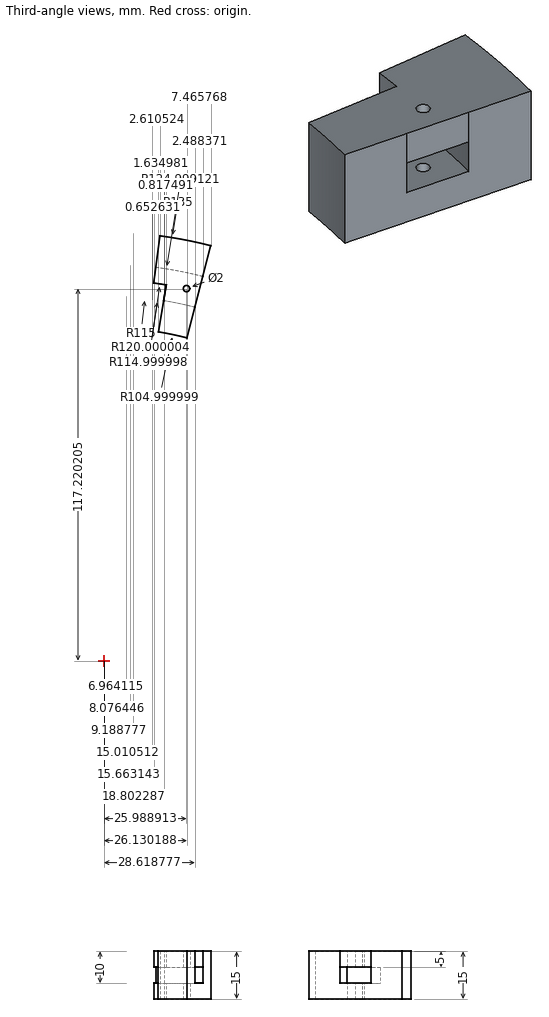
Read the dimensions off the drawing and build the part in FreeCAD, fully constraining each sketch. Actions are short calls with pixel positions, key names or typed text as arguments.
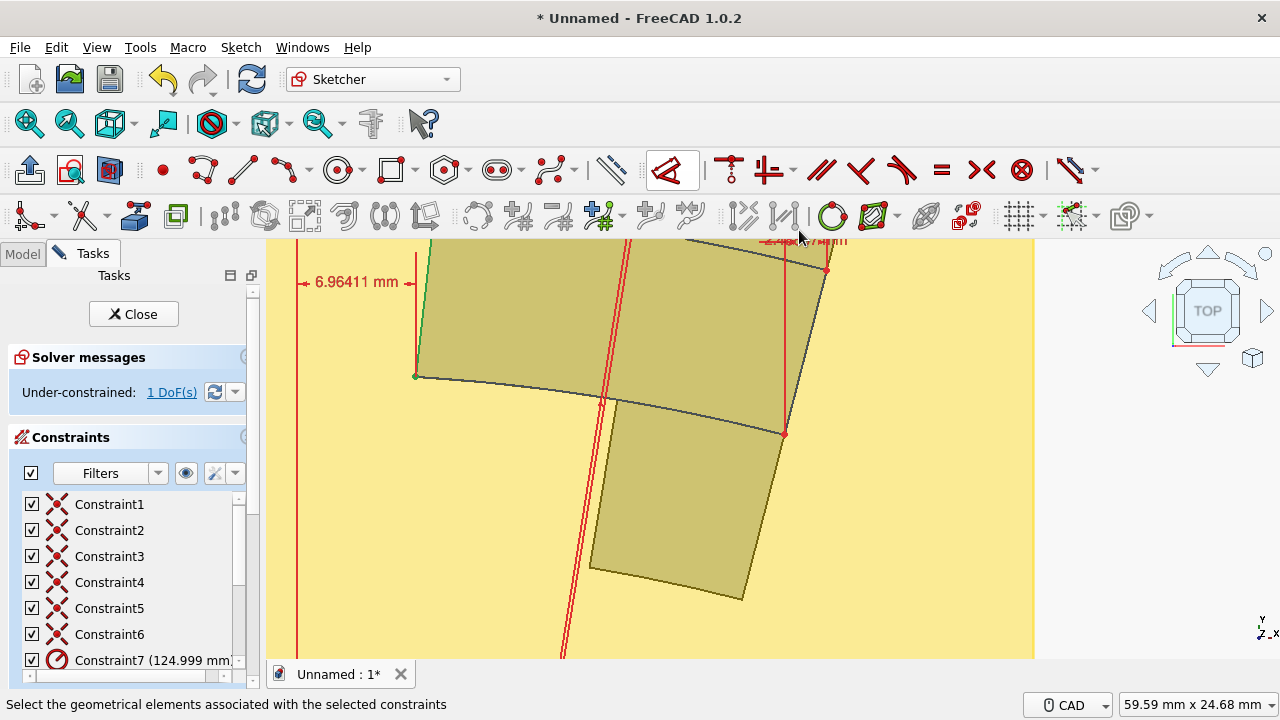
click(785, 435)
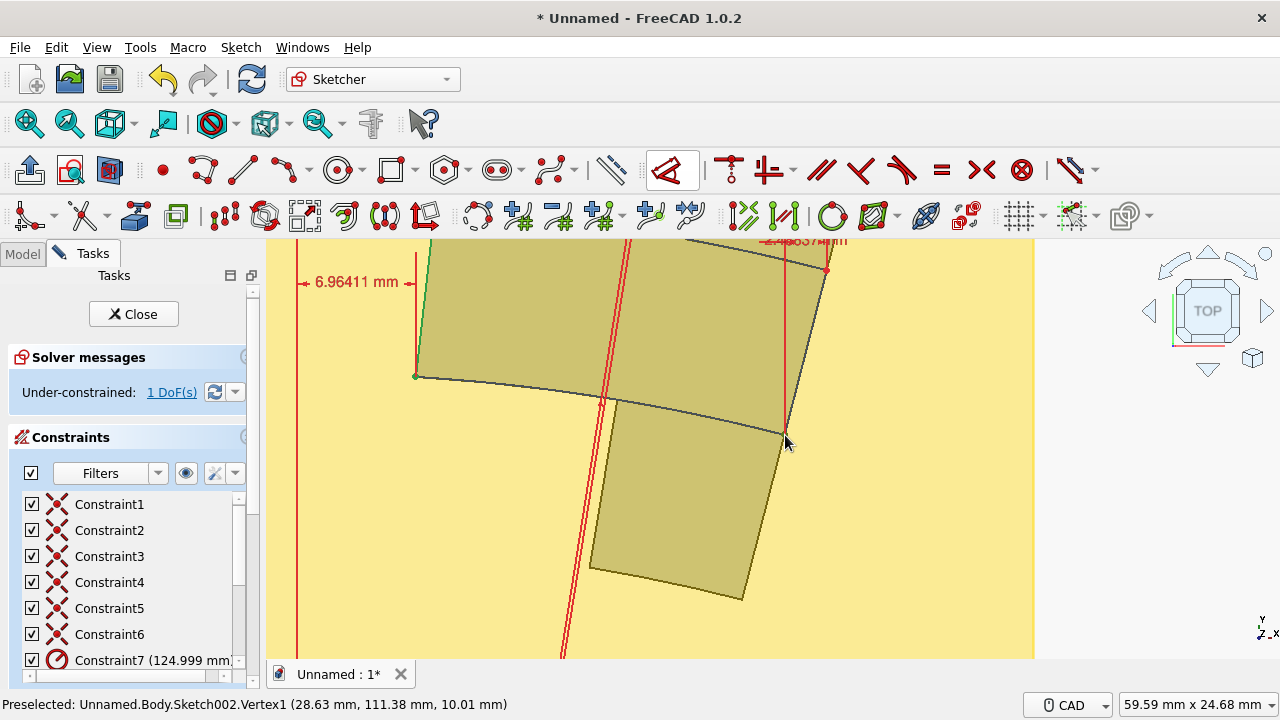
key(l)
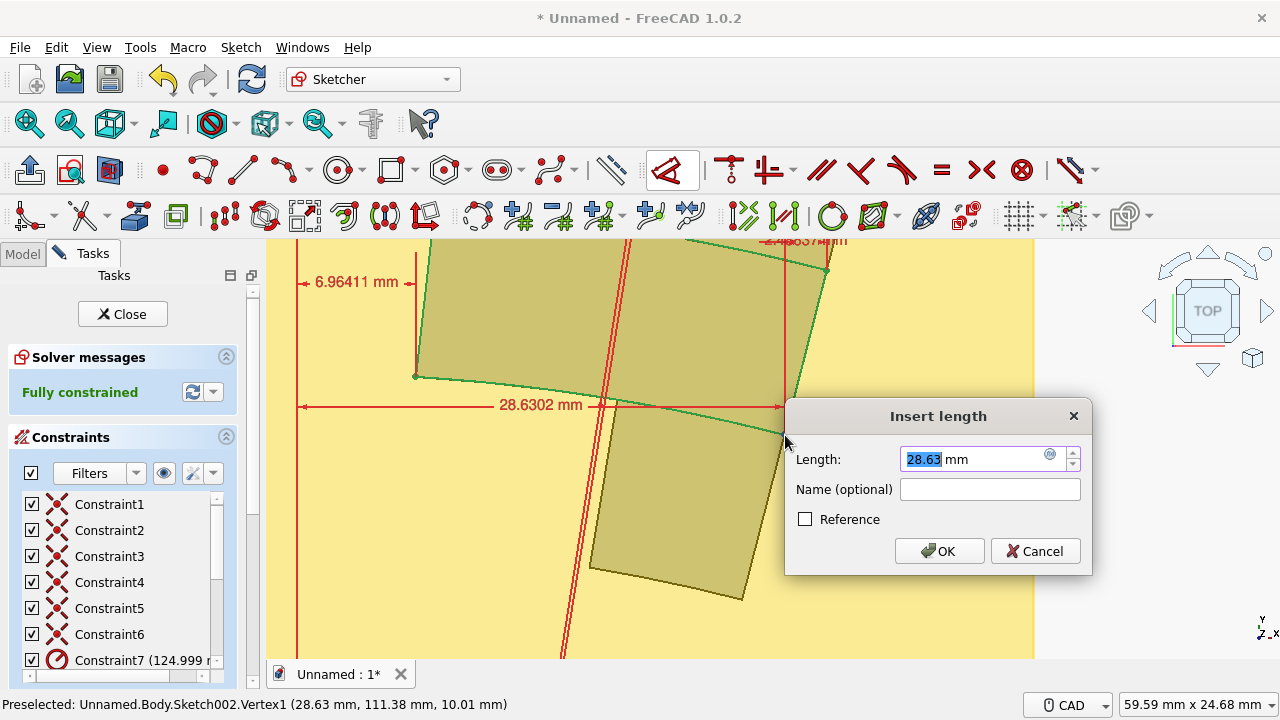
text(28.618777)
key(Return)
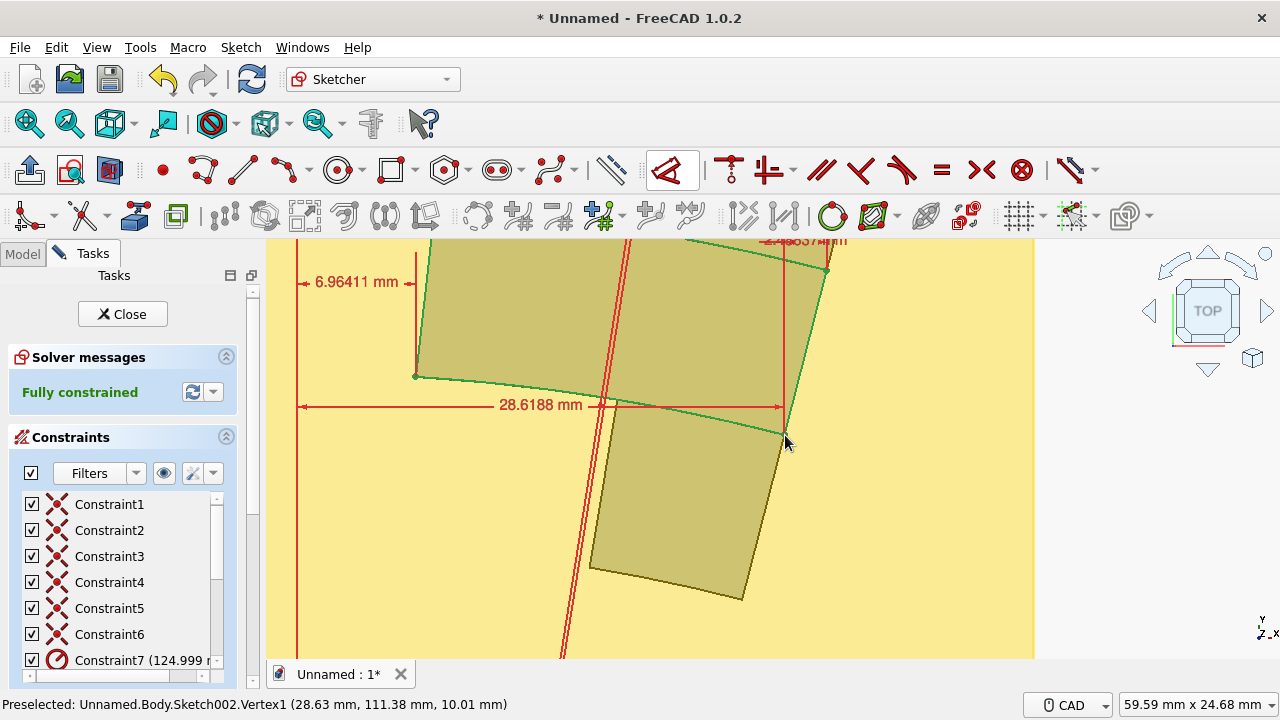
click(123, 314)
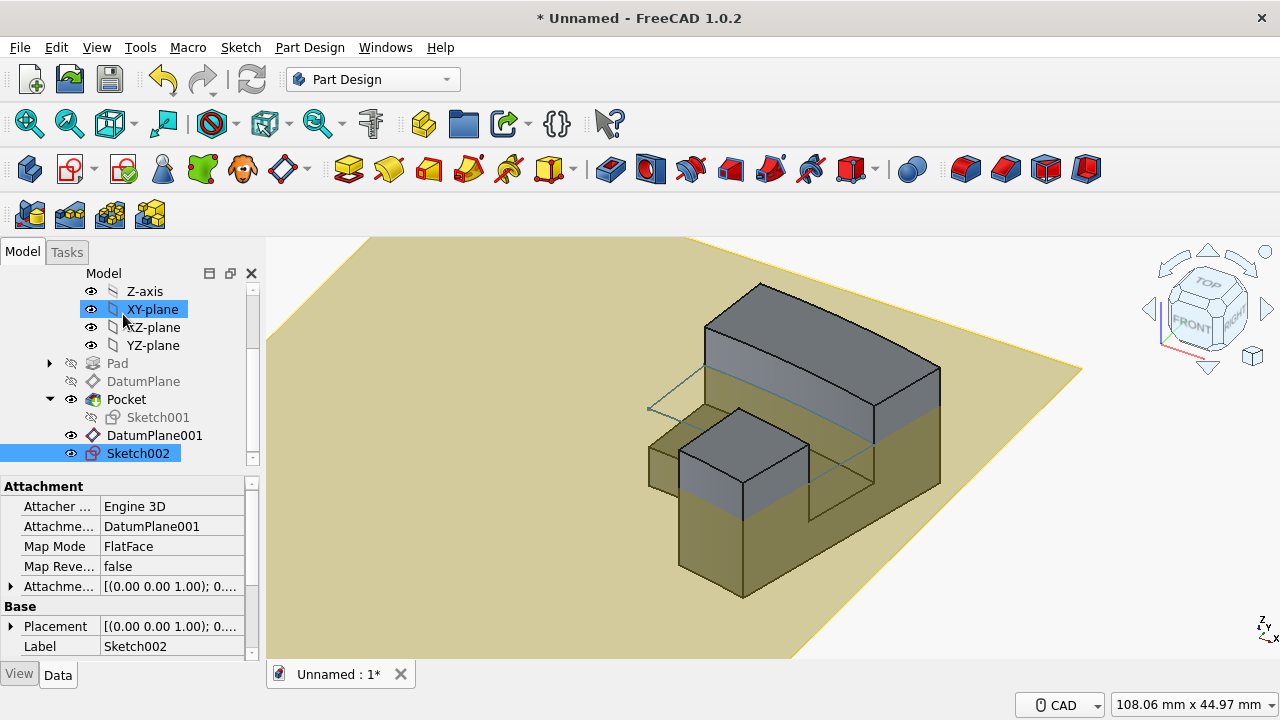
click(350, 170)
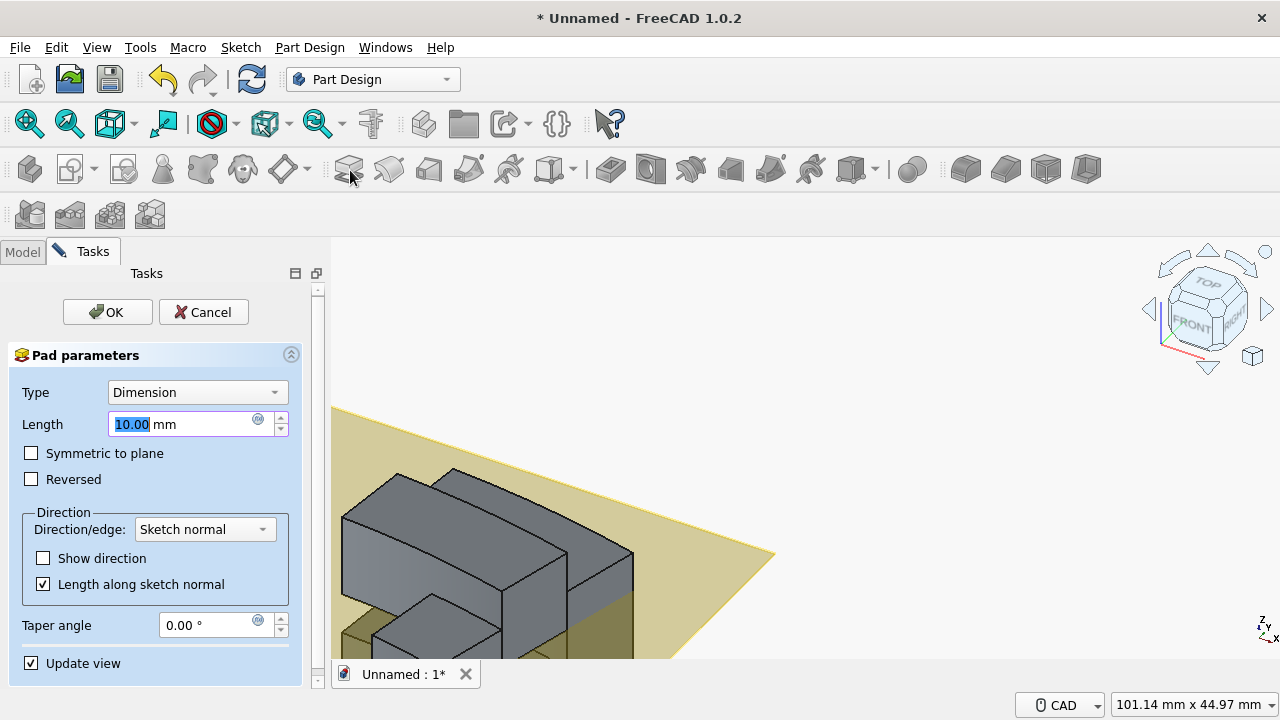
text(5)
key(Tab)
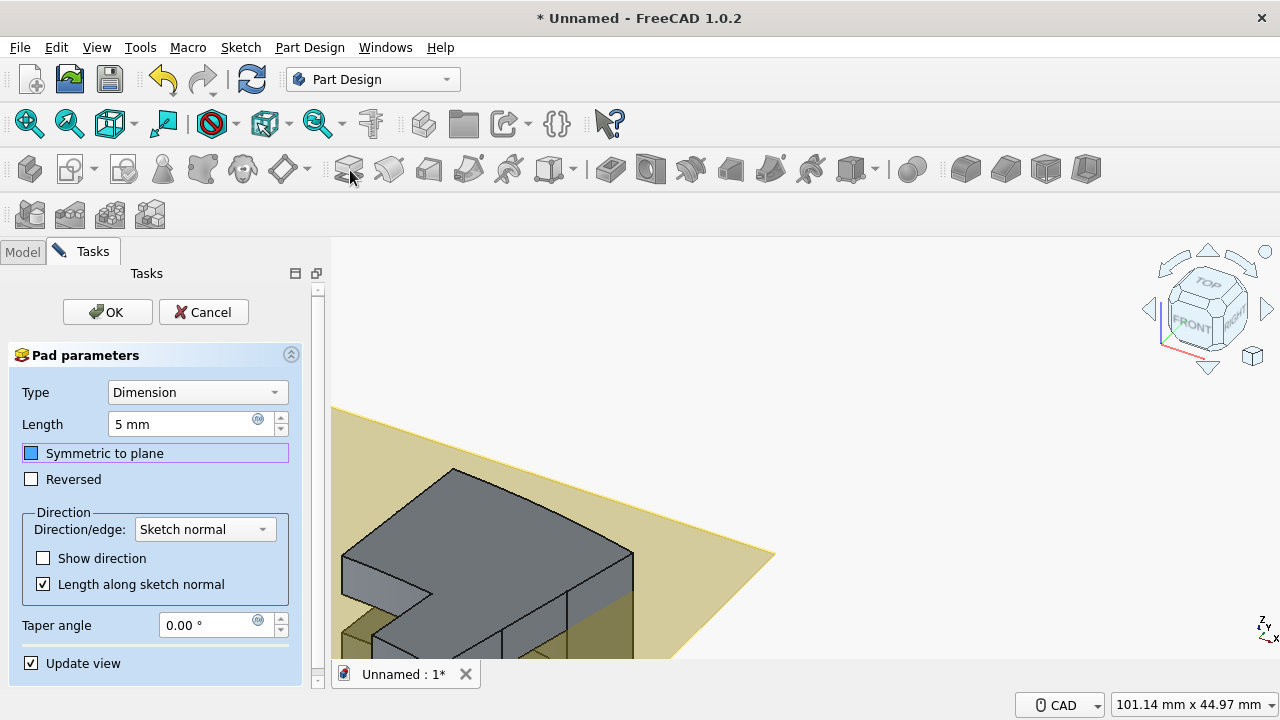
click(108, 312)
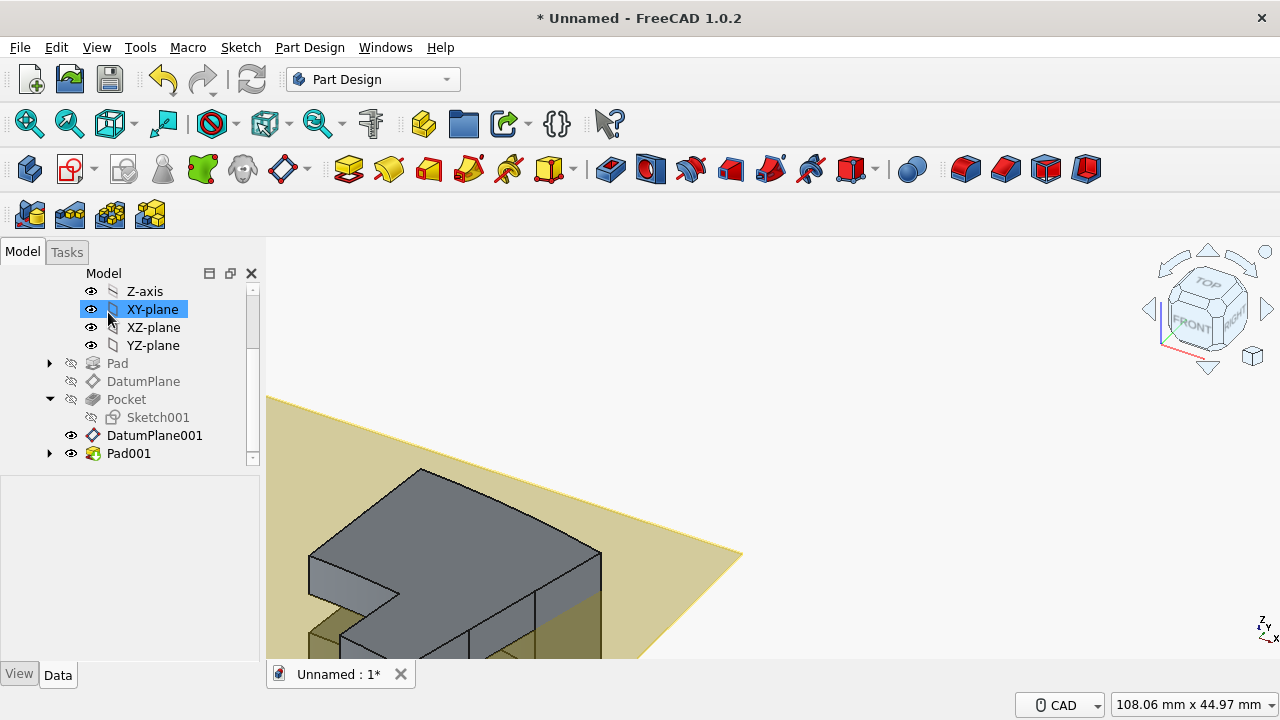
click(116, 435)
key(space)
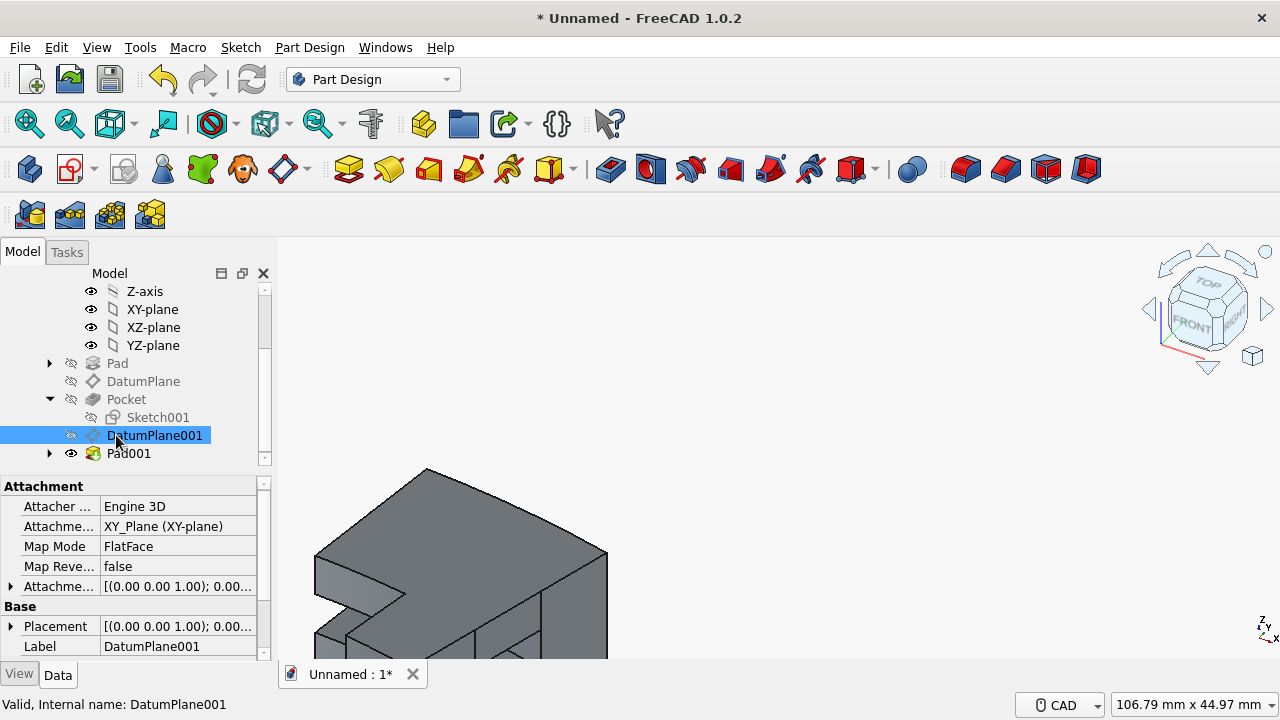
key(v)
key(f)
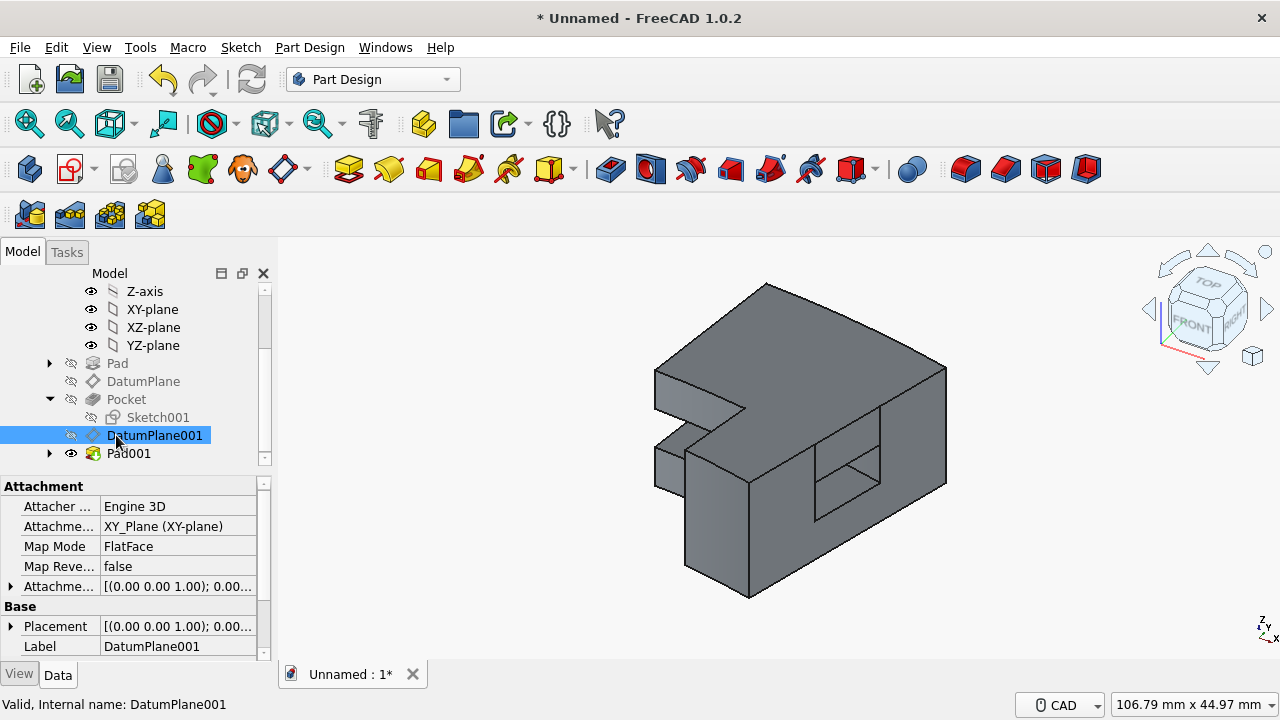
click(801, 367)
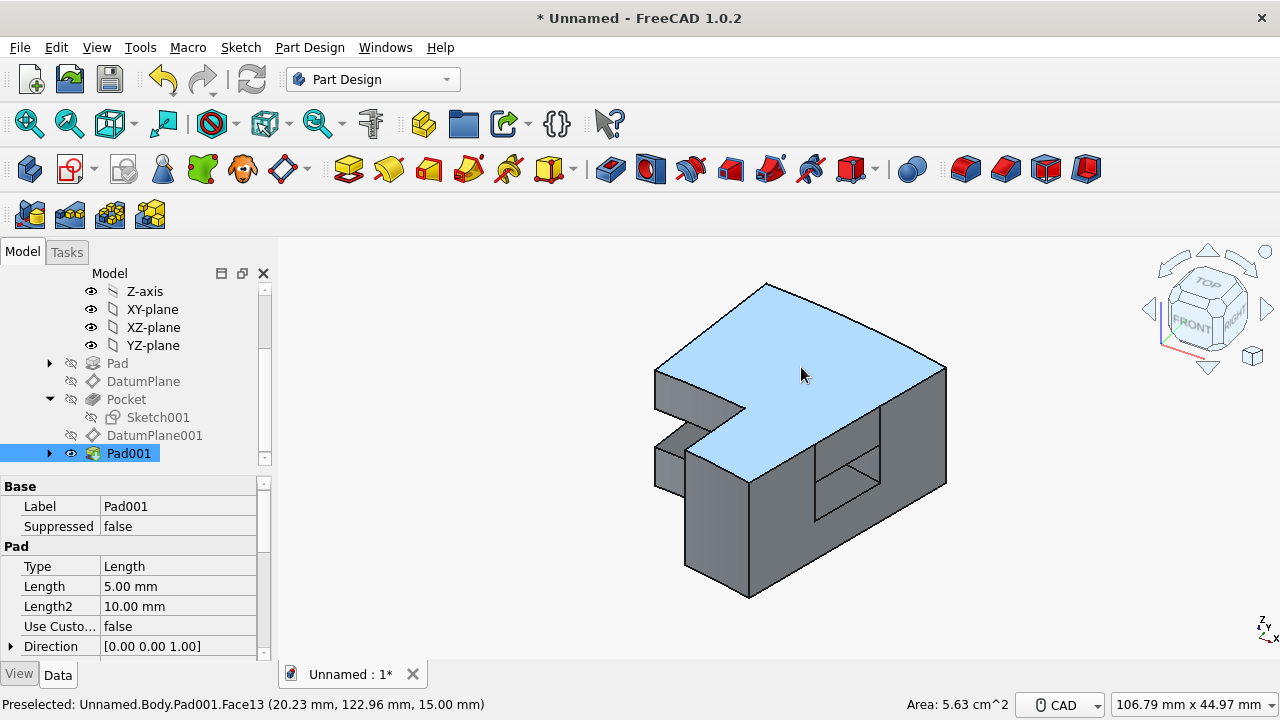
click(70, 170)